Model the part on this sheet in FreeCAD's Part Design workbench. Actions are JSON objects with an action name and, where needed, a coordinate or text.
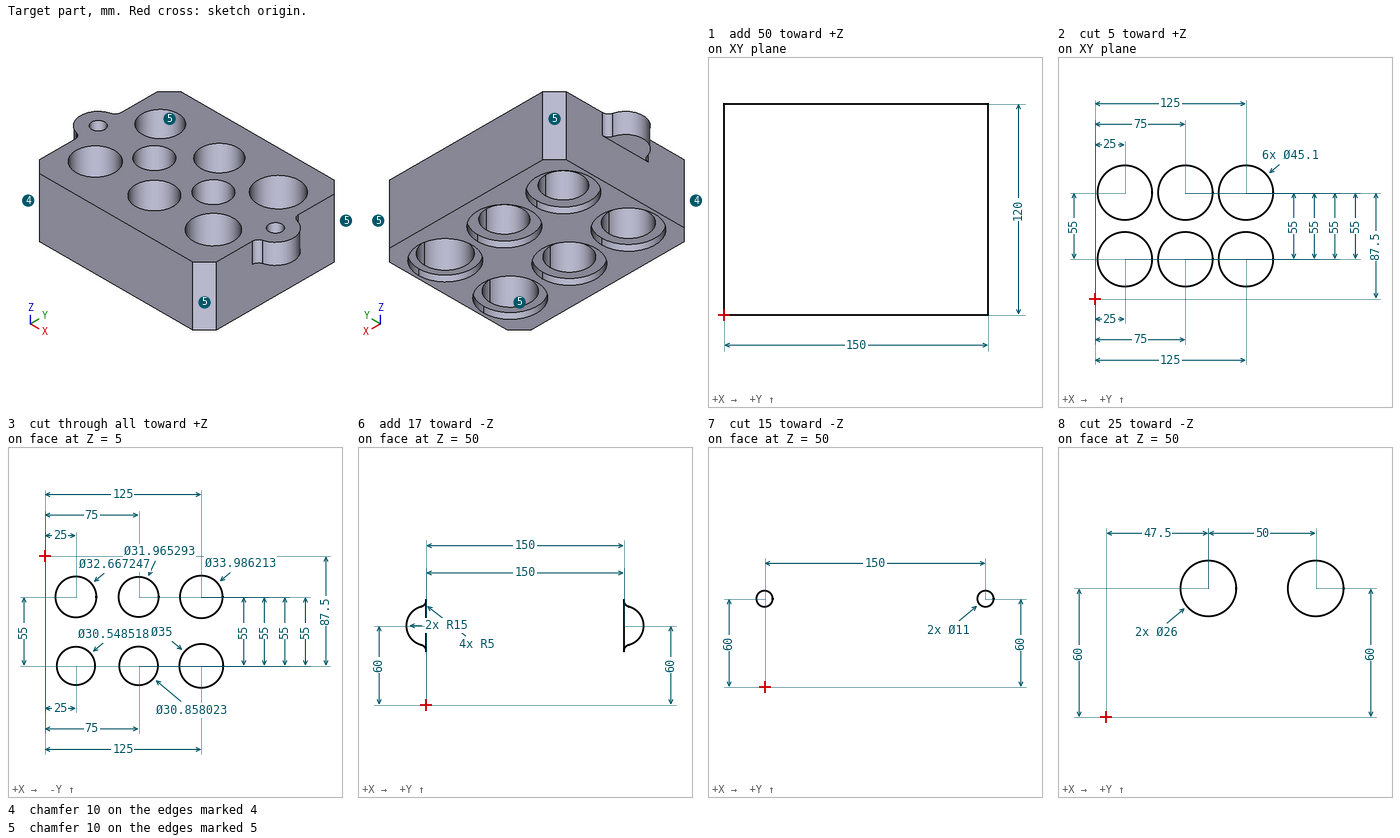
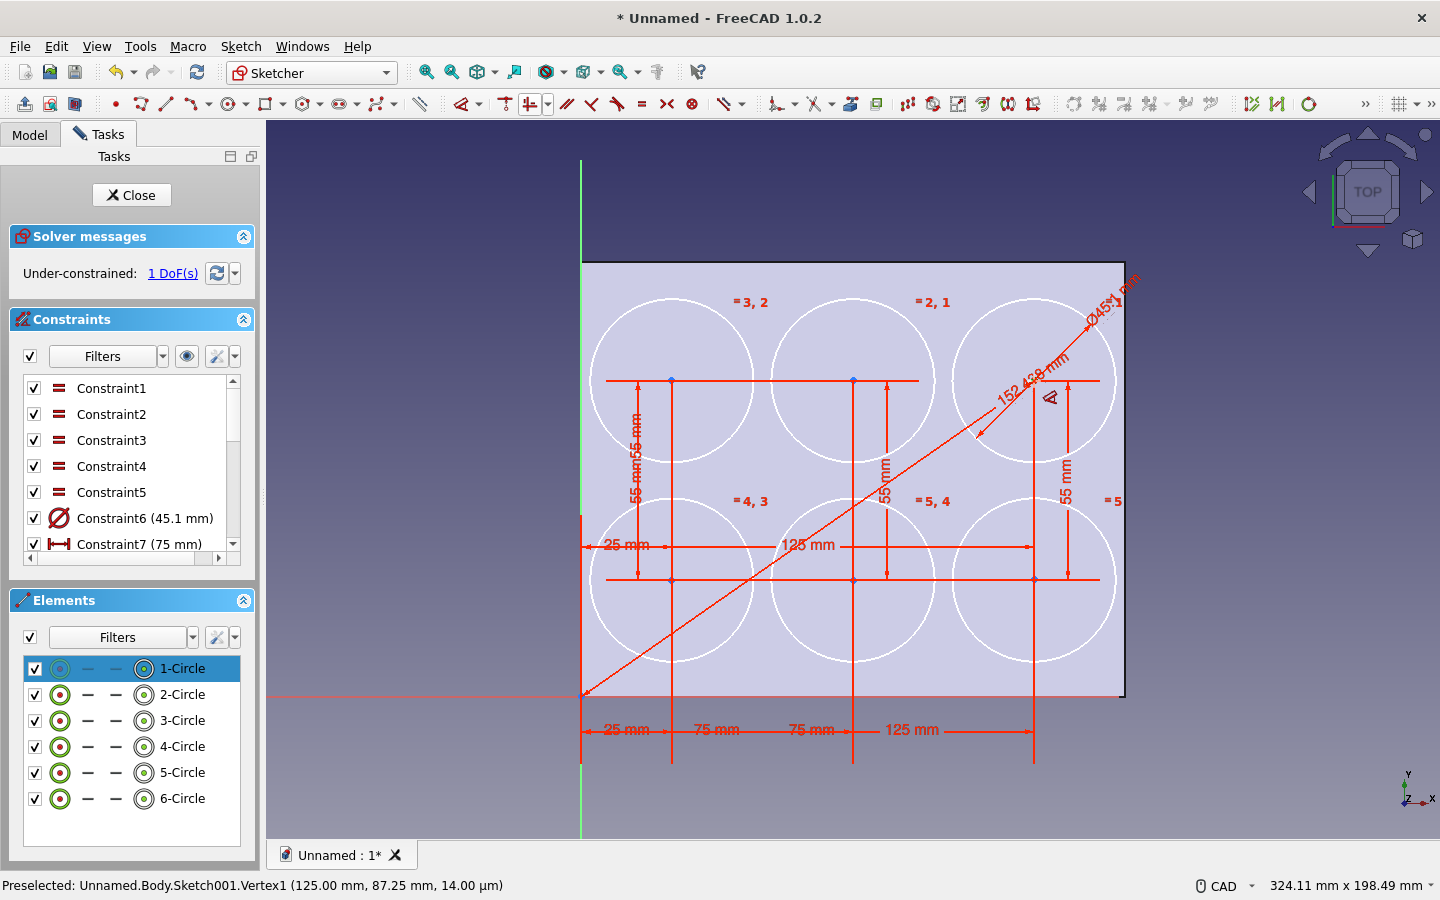
{"action": "left_click", "coordinate": [1034, 580]}
{"action": "left_click", "coordinate": [1068, 435]}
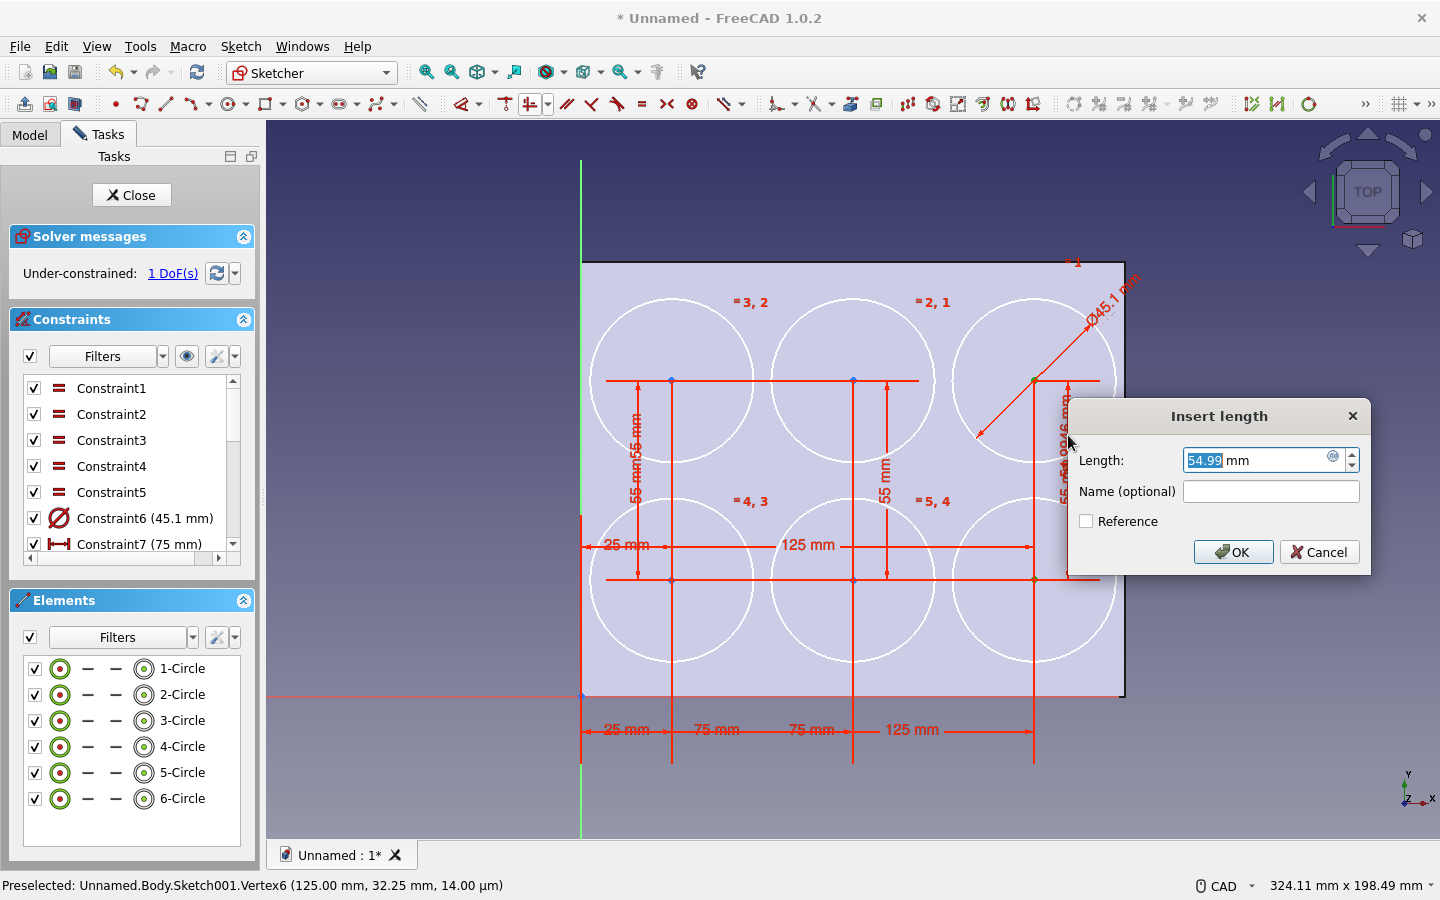
{"action": "type", "text": "55"}
{"action": "key", "text": "Return"}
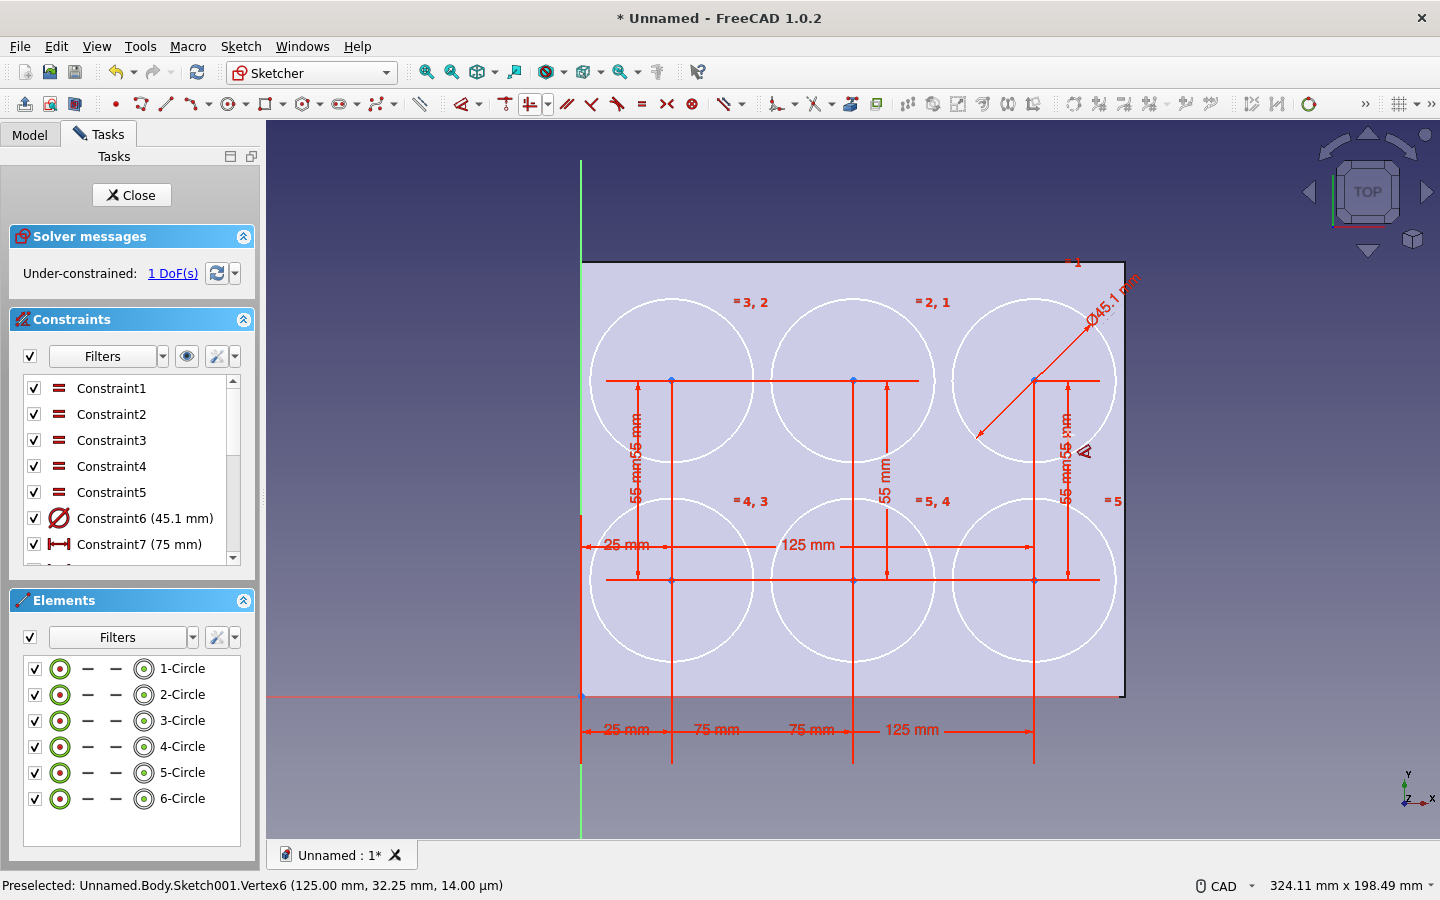
{"action": "left_click", "coordinate": [1034, 381]}
{"action": "left_click", "coordinate": [547, 539]}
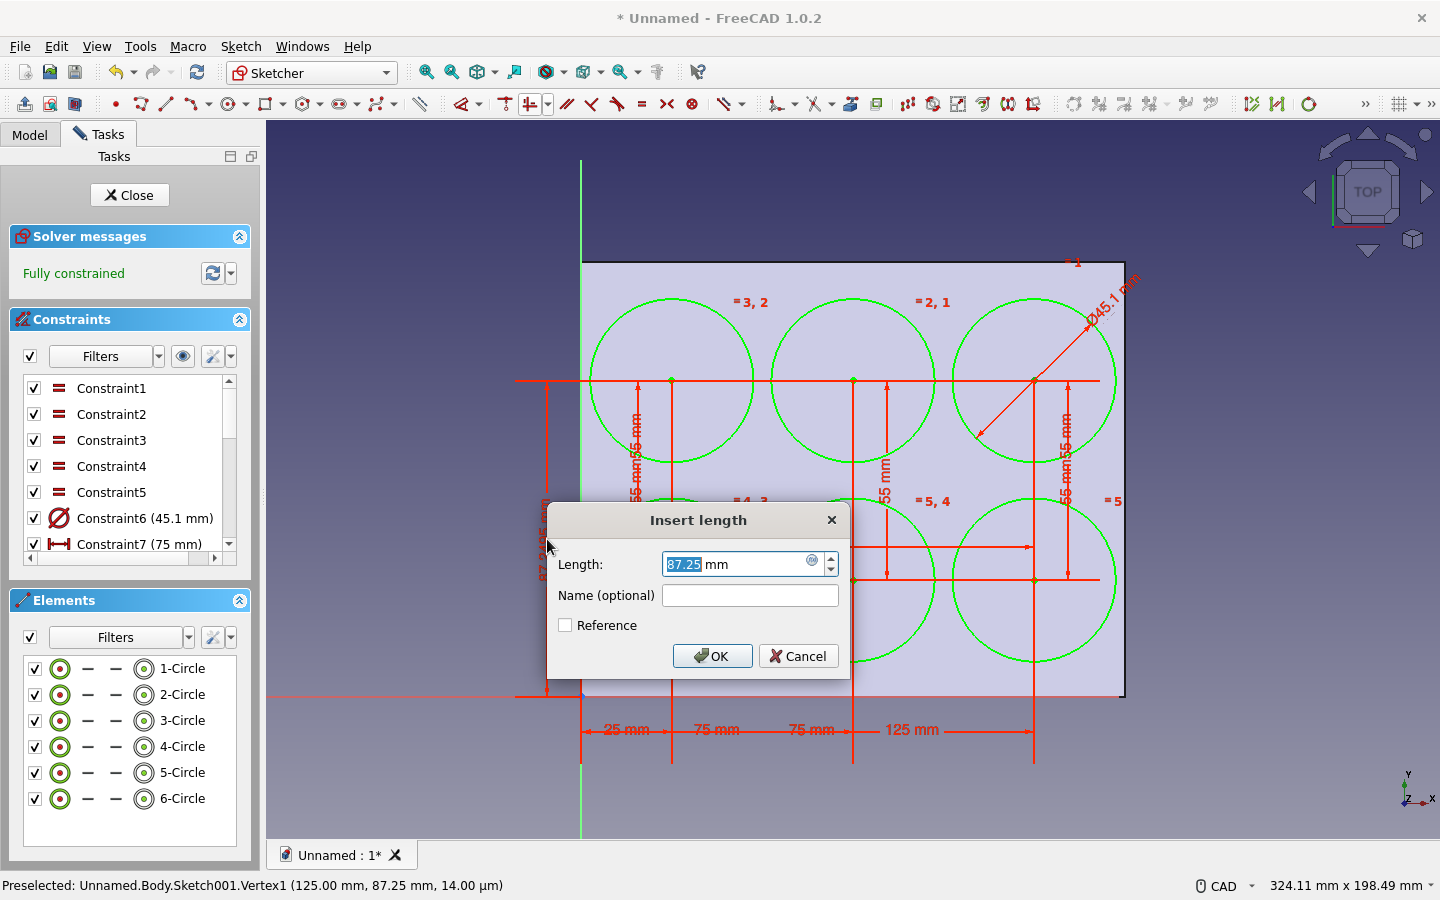
{"action": "type", "text": "87.5"}
{"action": "key", "text": "Return"}
{"action": "key", "text": "Escape"}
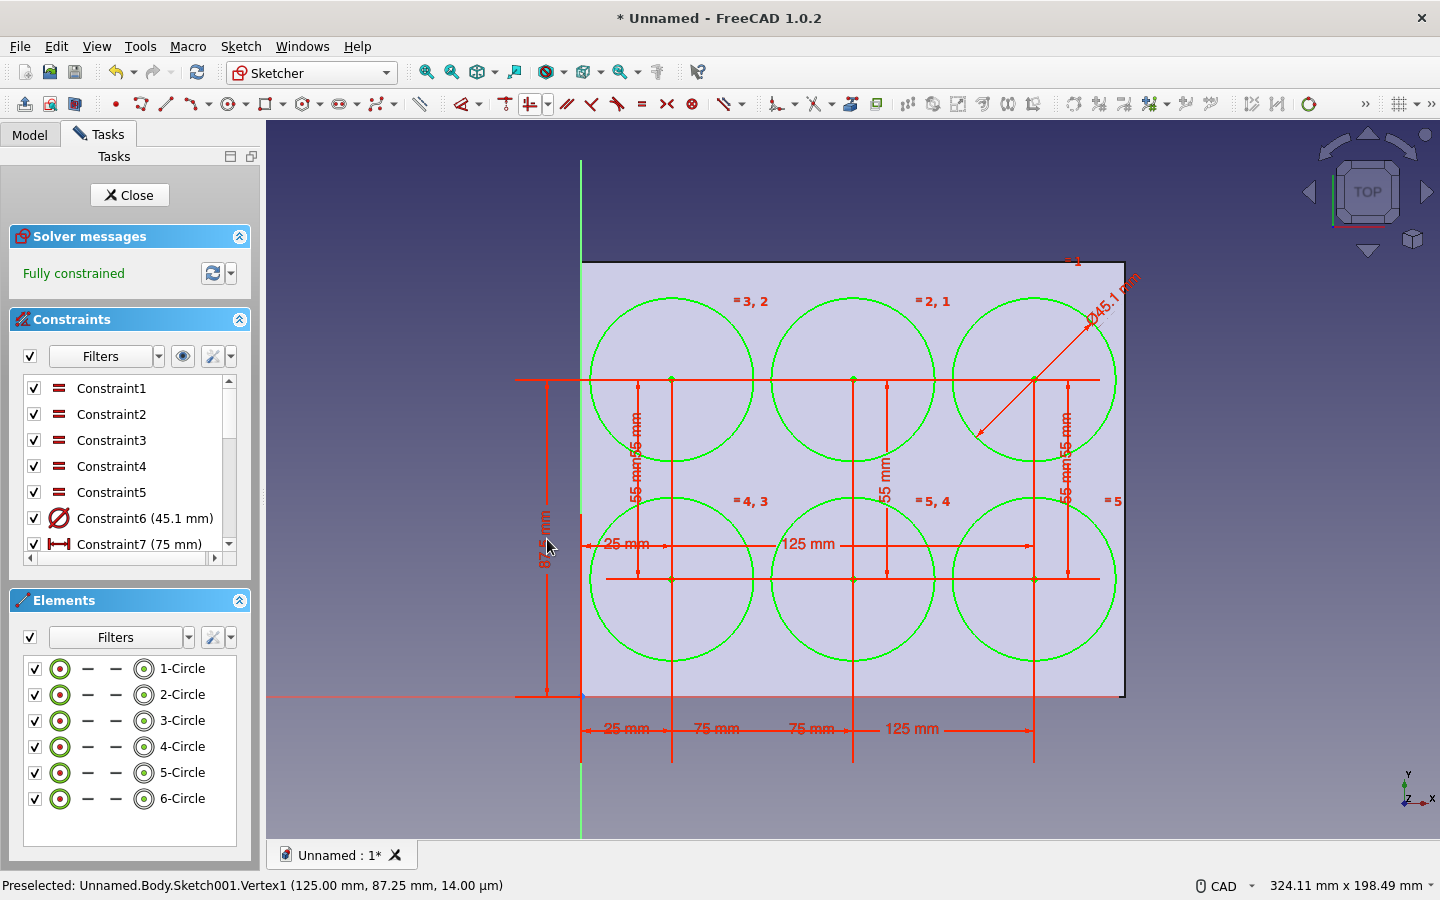
{"action": "left_click", "coordinate": [130, 195]}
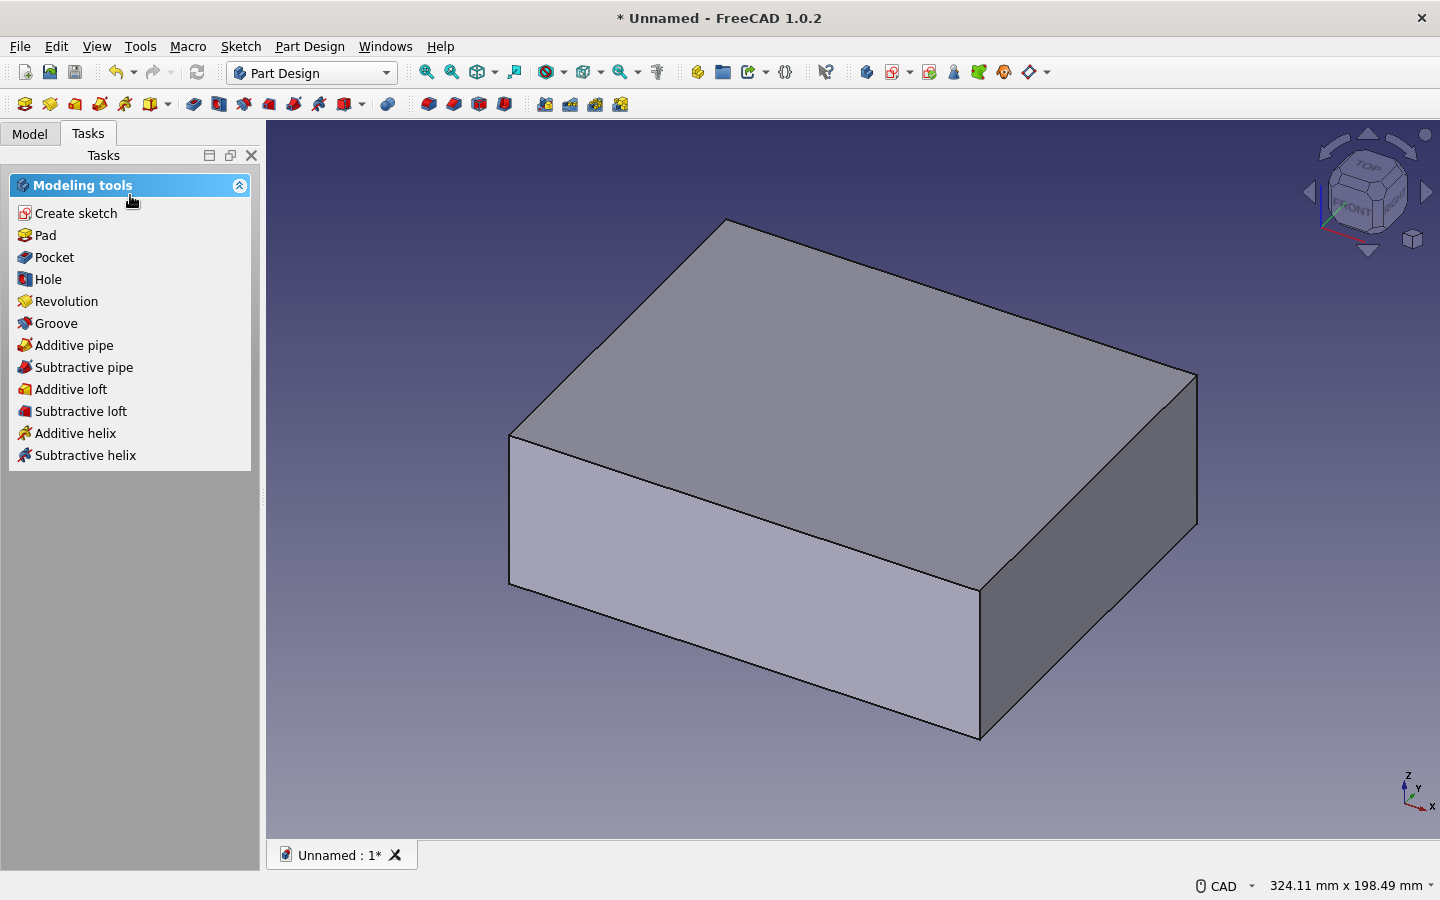
{"action": "left_click", "coordinate": [194, 104]}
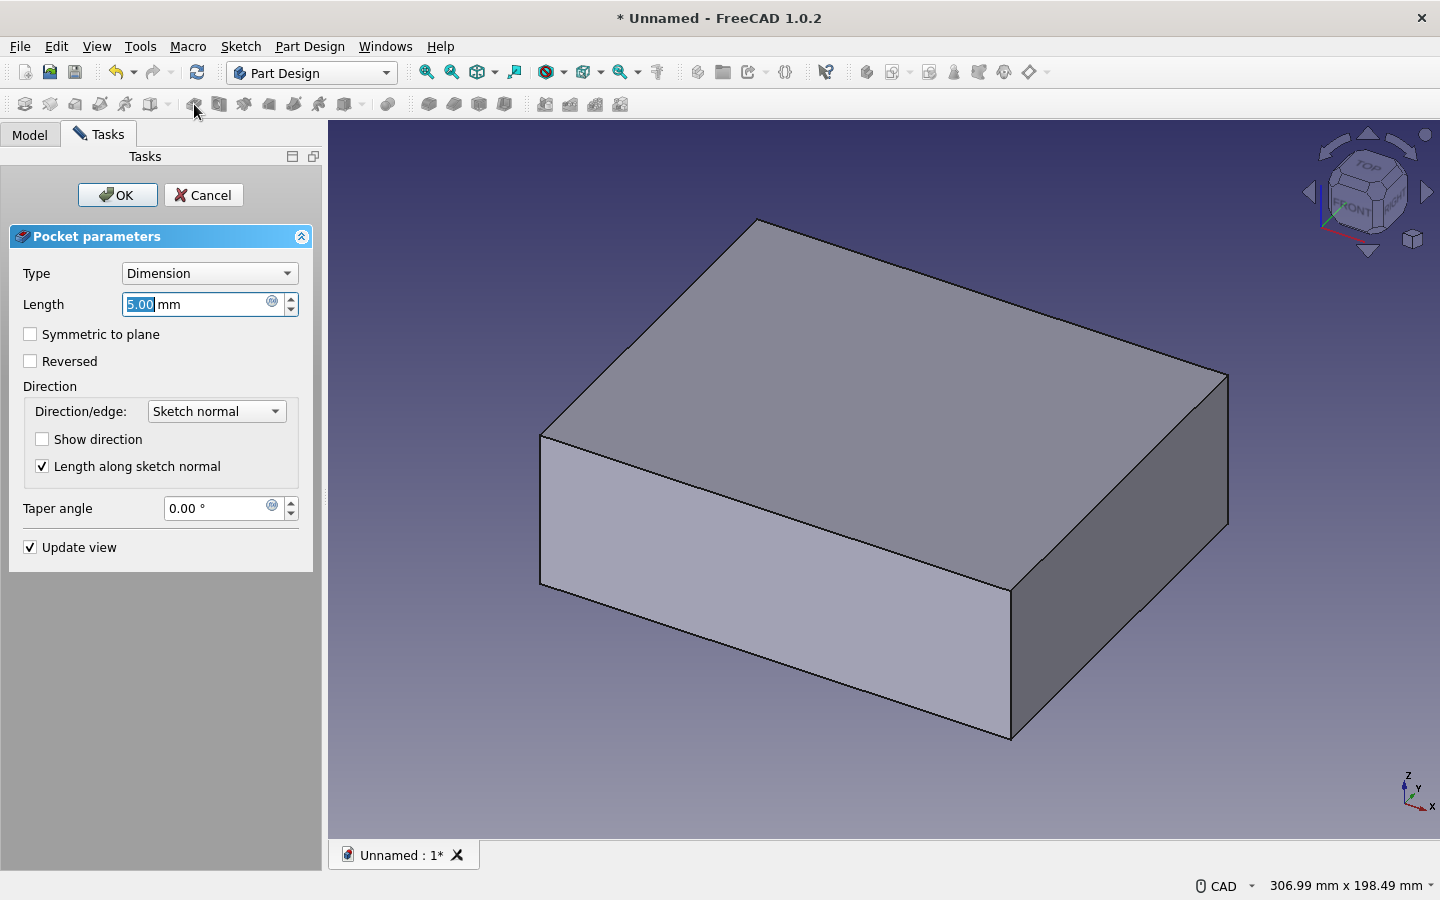
{"action": "type", "text": "5"}
{"action": "key", "text": "Tab"}